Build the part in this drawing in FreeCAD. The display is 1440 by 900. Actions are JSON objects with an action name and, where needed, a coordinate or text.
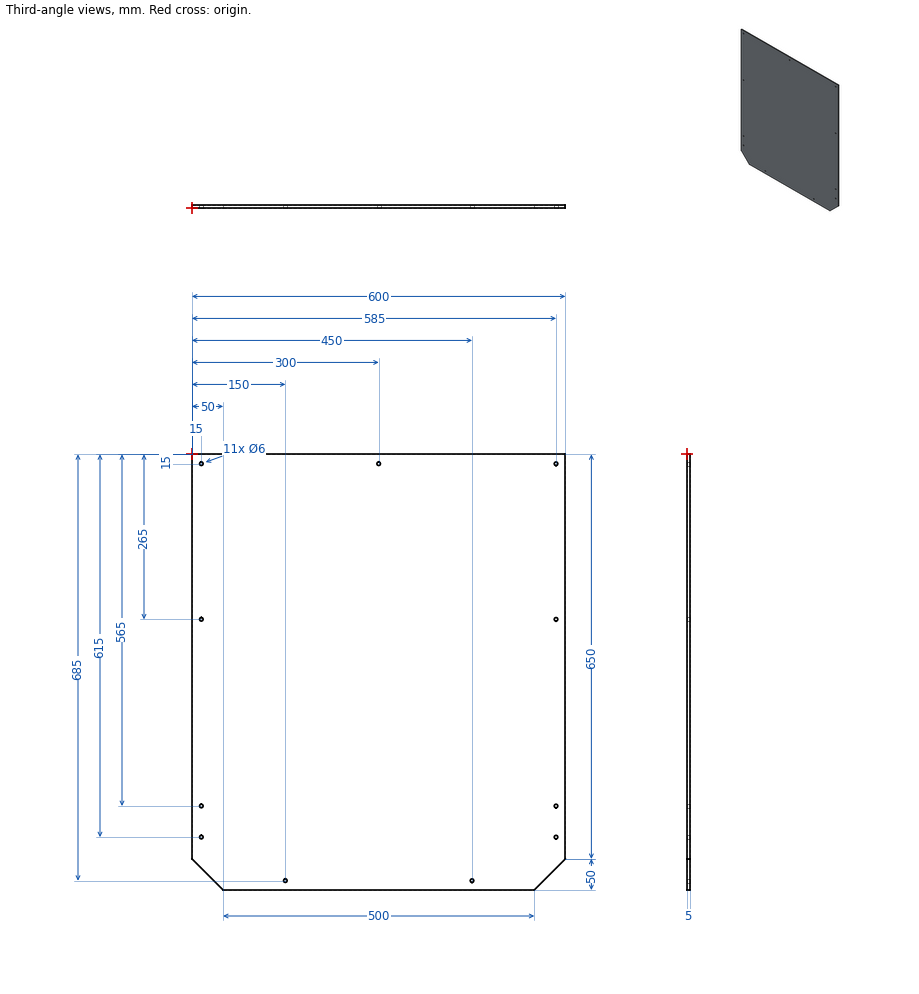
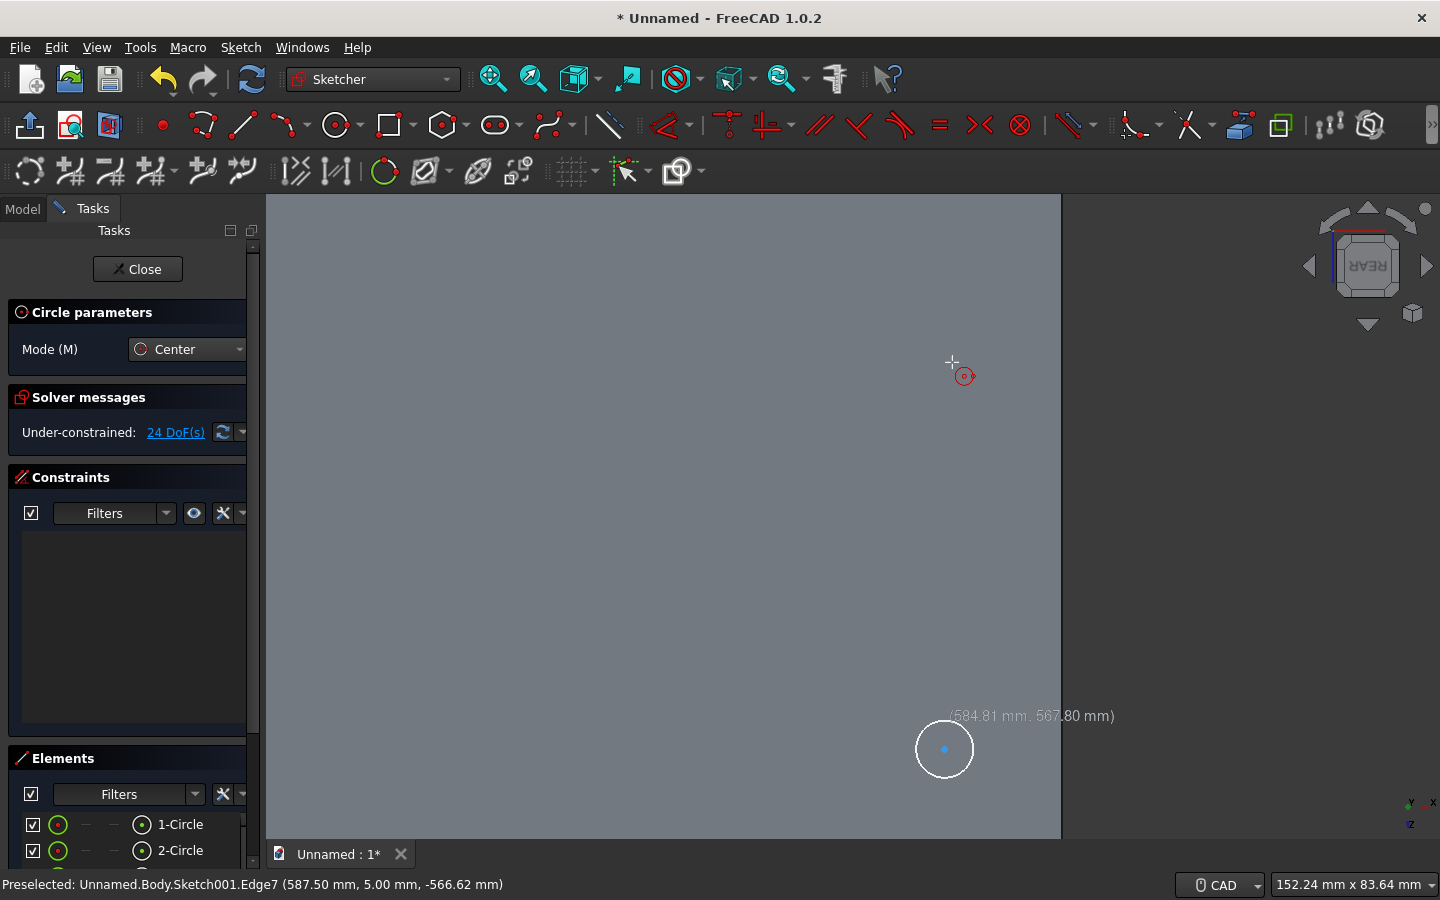
{"action": "scroll", "coordinate": [952, 362], "scroll_direction": "down", "scroll_amount": 13}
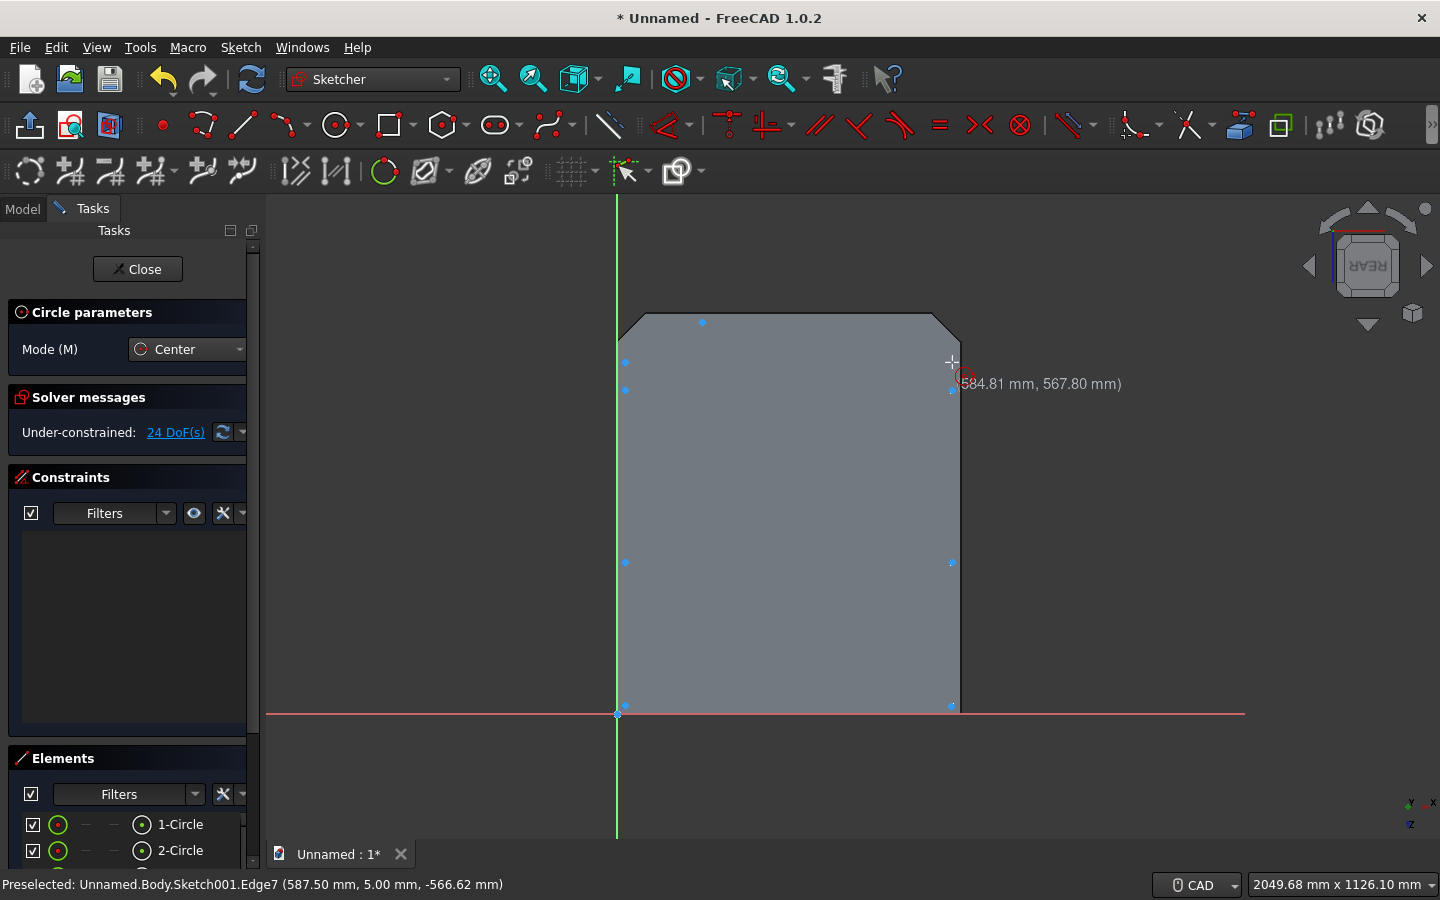
{"action": "left_click", "coordinate": [952, 362]}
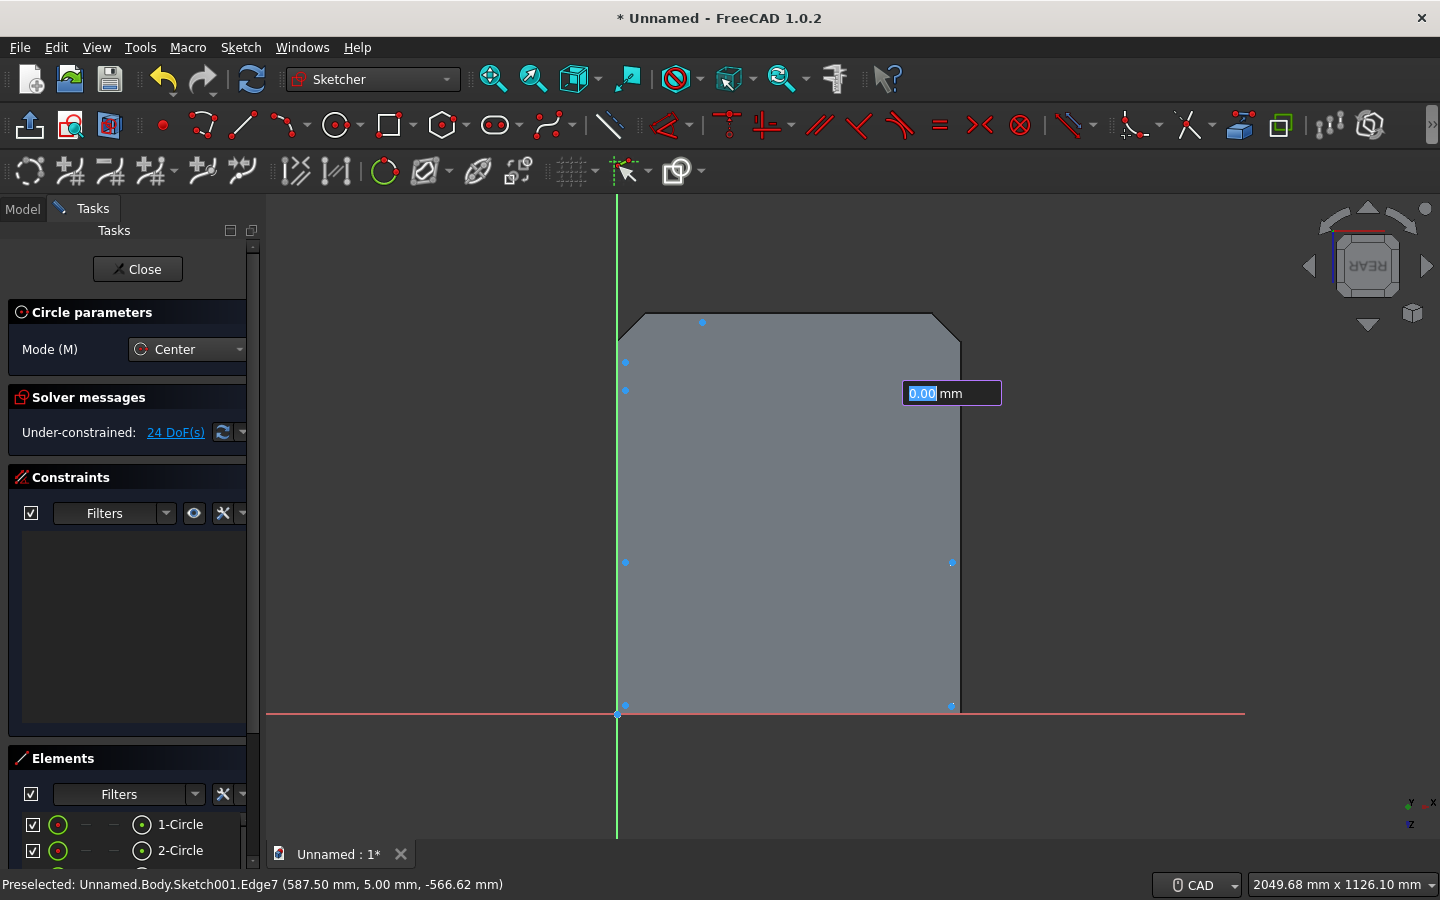
{"action": "scroll", "coordinate": [953, 361], "scroll_direction": "up", "scroll_amount": 12}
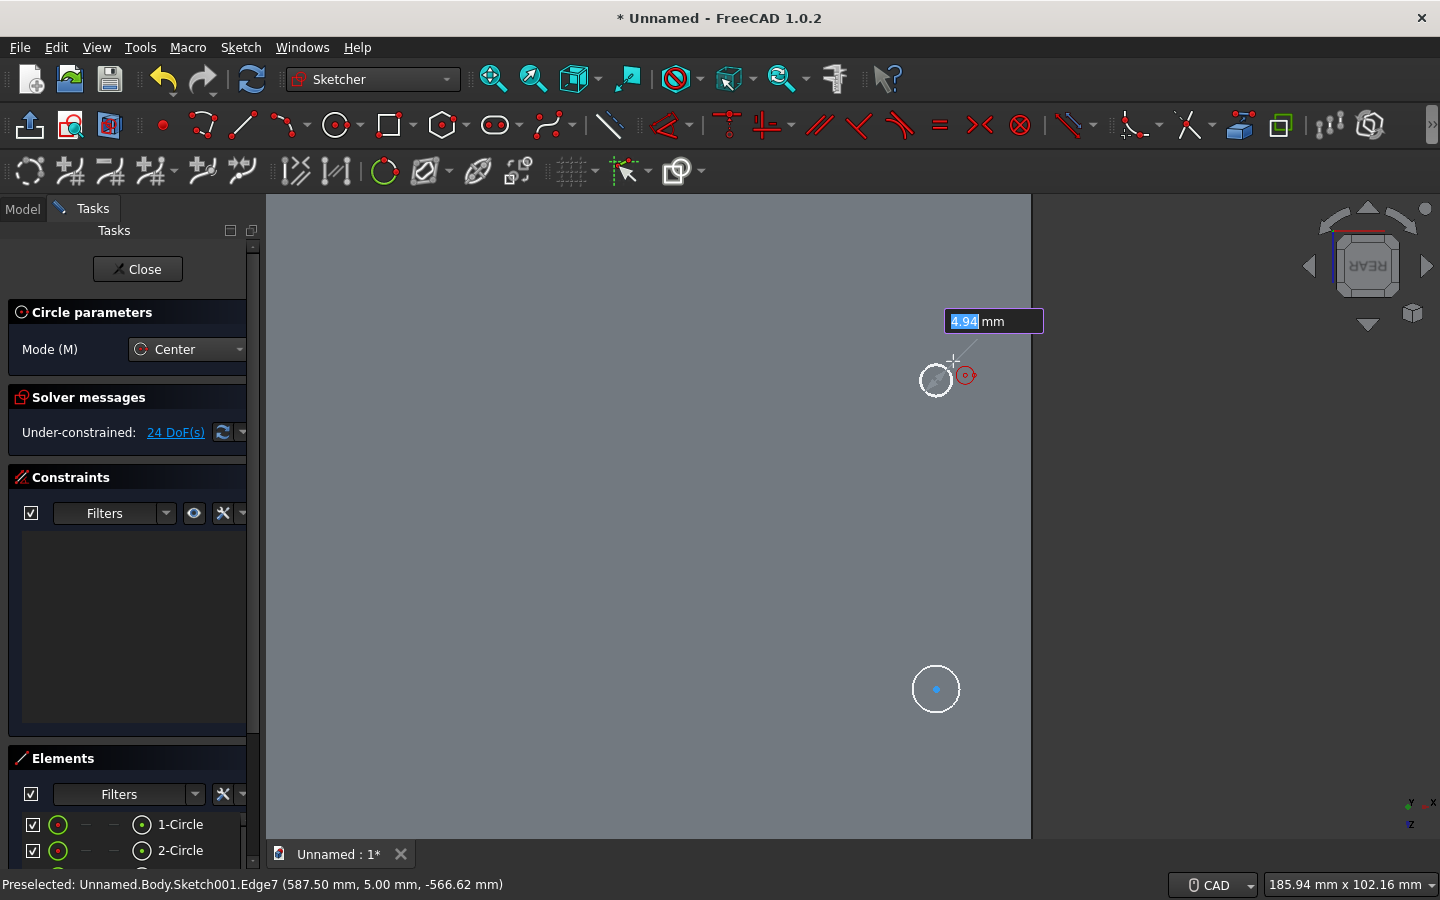
{"action": "left_click", "coordinate": [951, 354]}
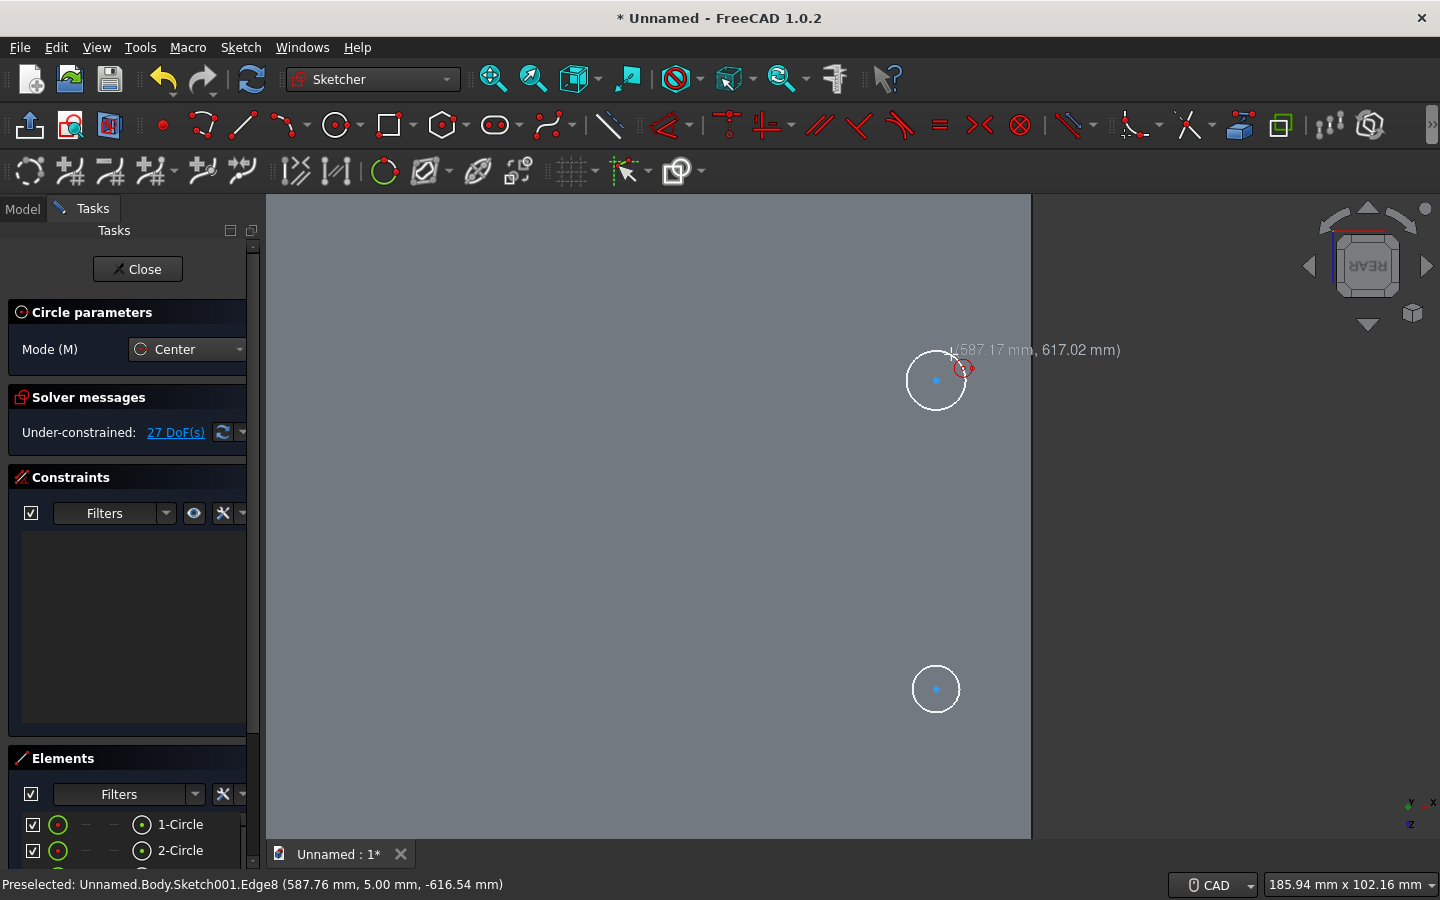
{"action": "scroll", "coordinate": [953, 361], "scroll_direction": "down", "scroll_amount": 12}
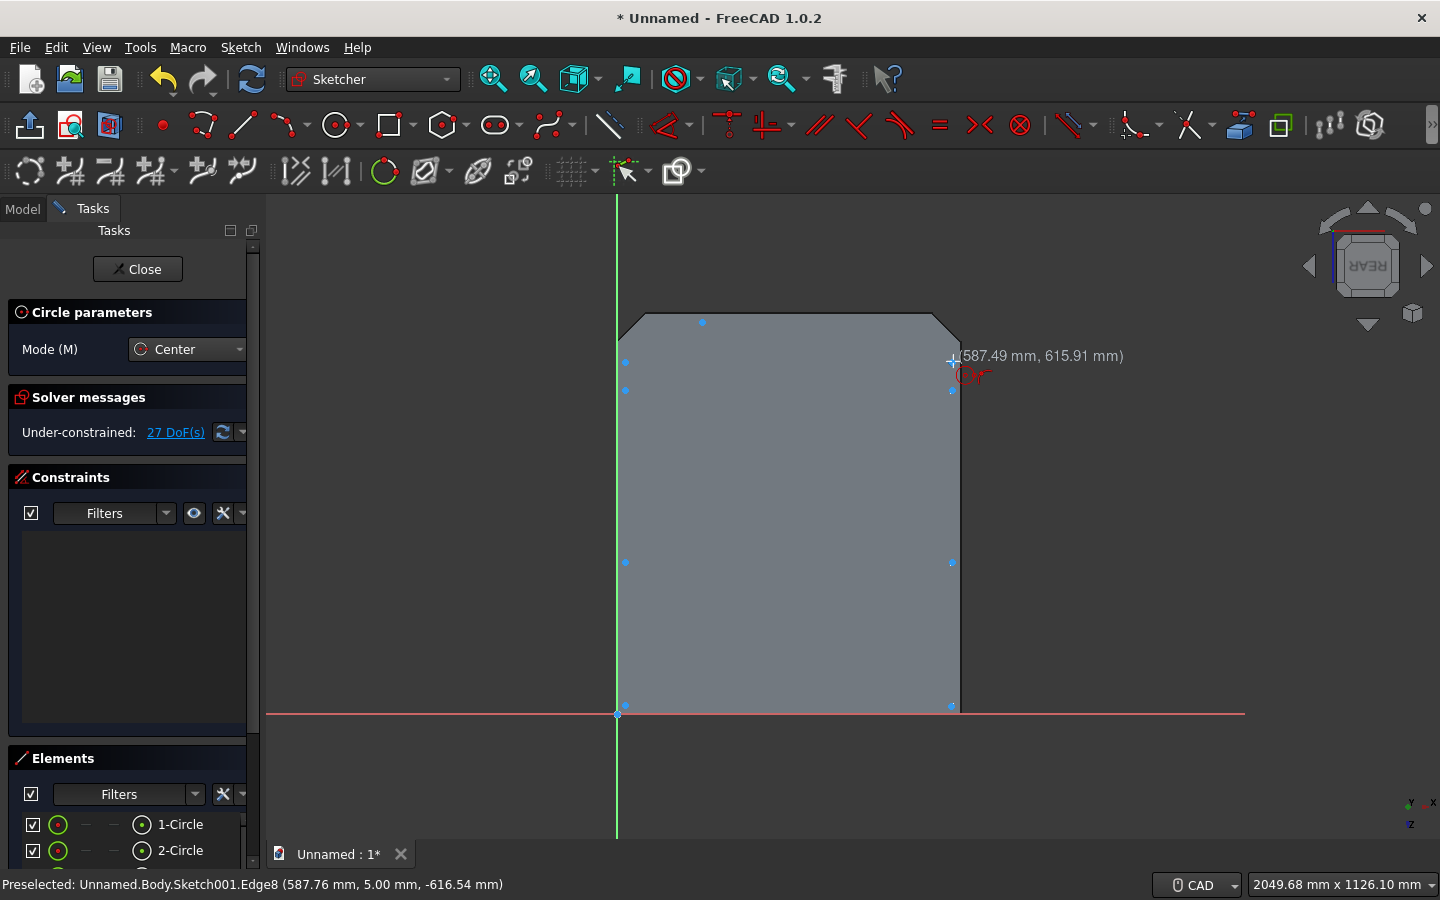
{"action": "scroll", "coordinate": [875, 322], "scroll_direction": "up", "scroll_amount": 13}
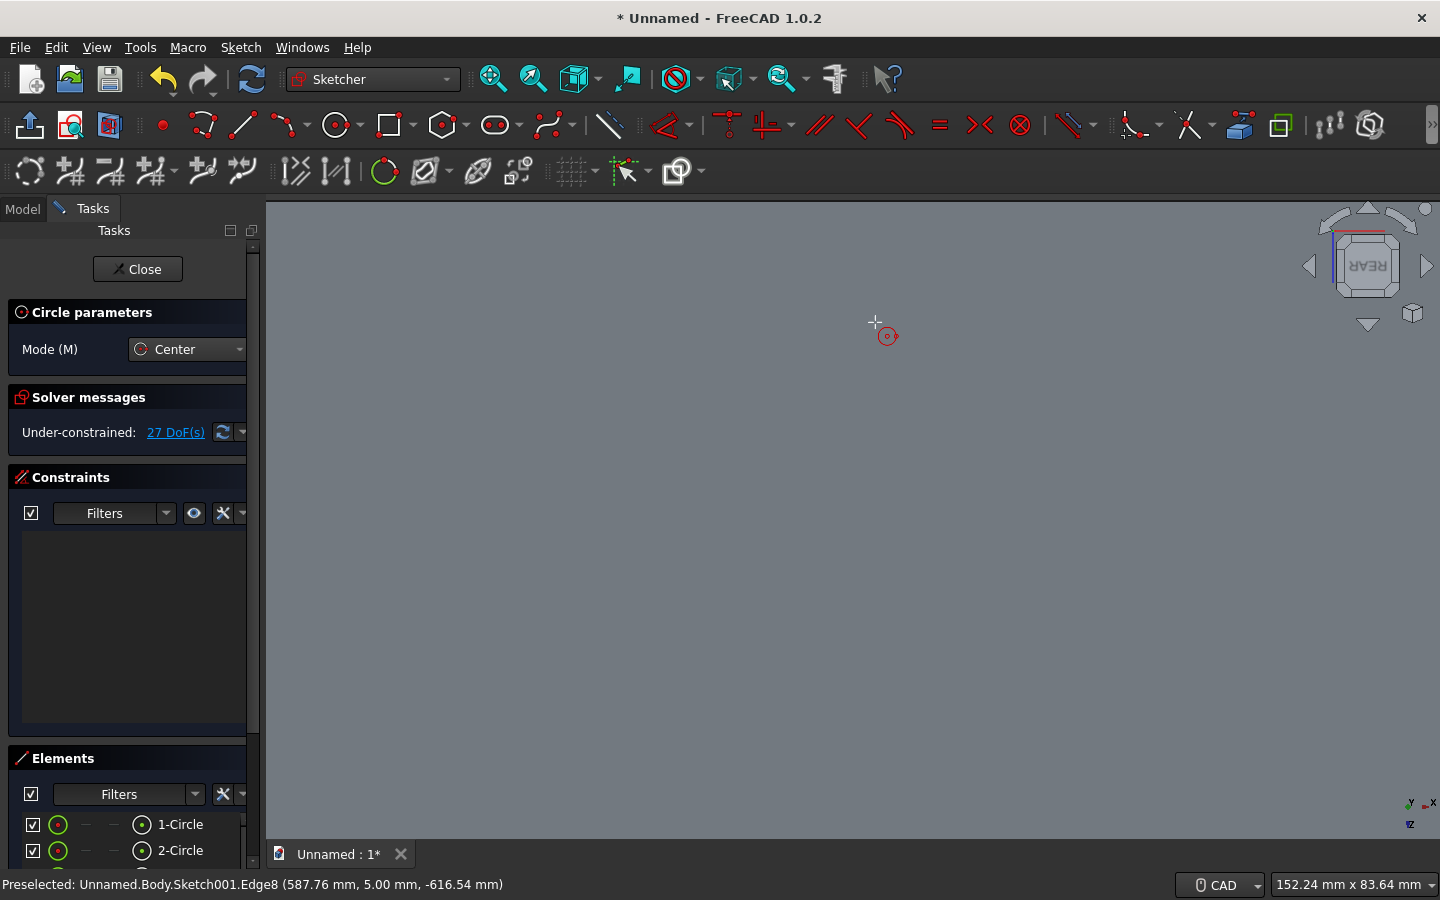
{"action": "scroll", "coordinate": [875, 322], "scroll_direction": "down", "scroll_amount": 13}